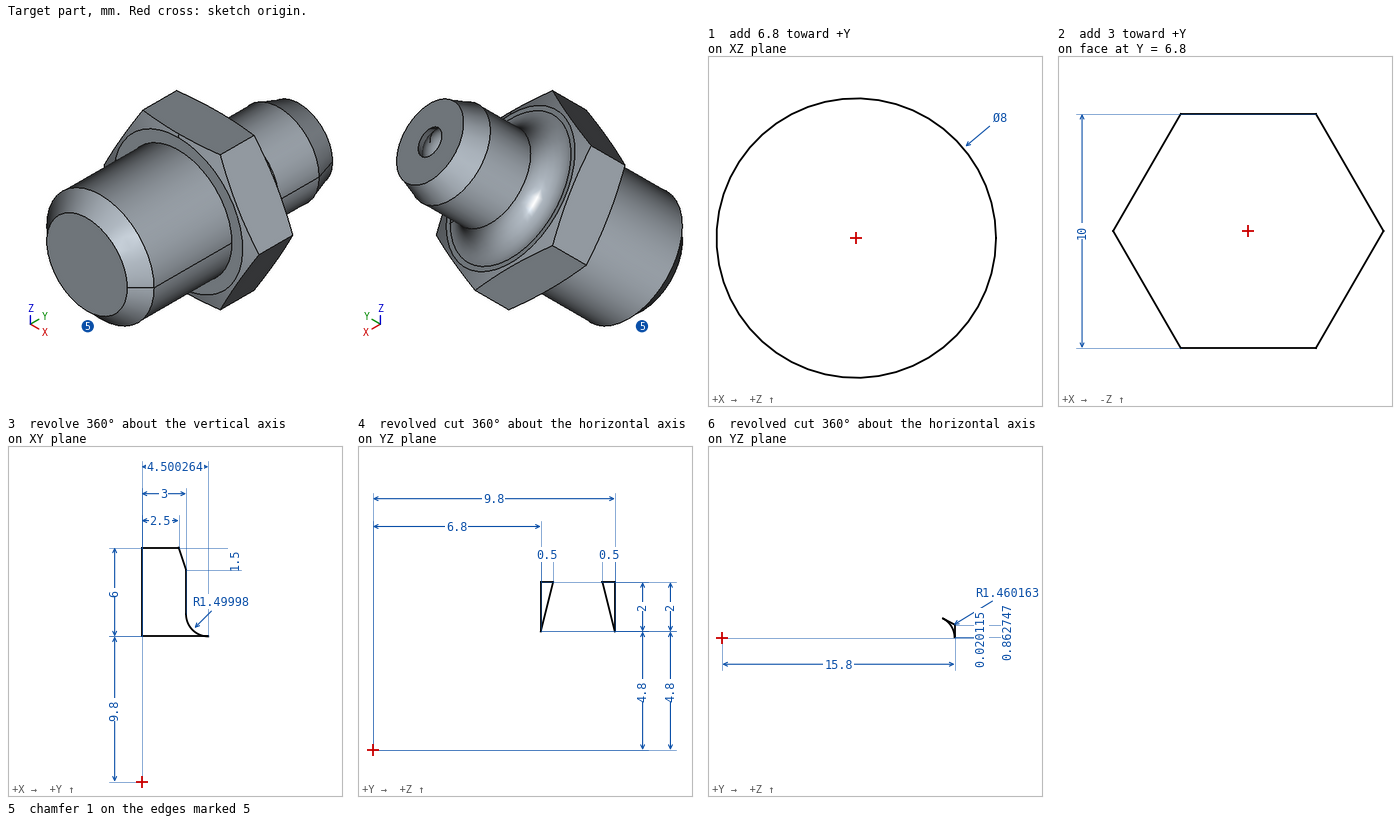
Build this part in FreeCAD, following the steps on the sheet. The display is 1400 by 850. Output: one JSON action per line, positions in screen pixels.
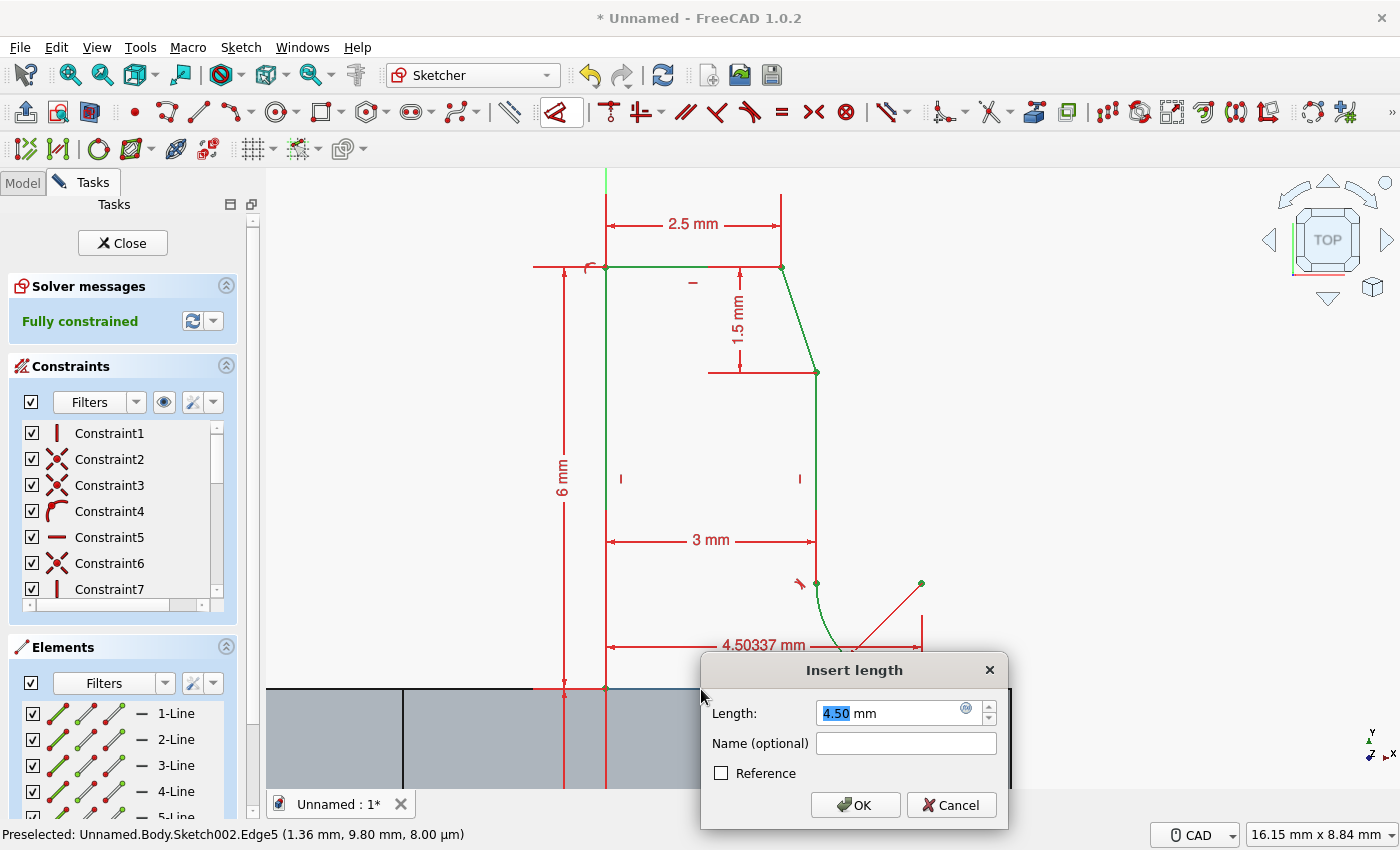
{"action": "type", "text": "4.500264"}
{"action": "key", "text": "Return"}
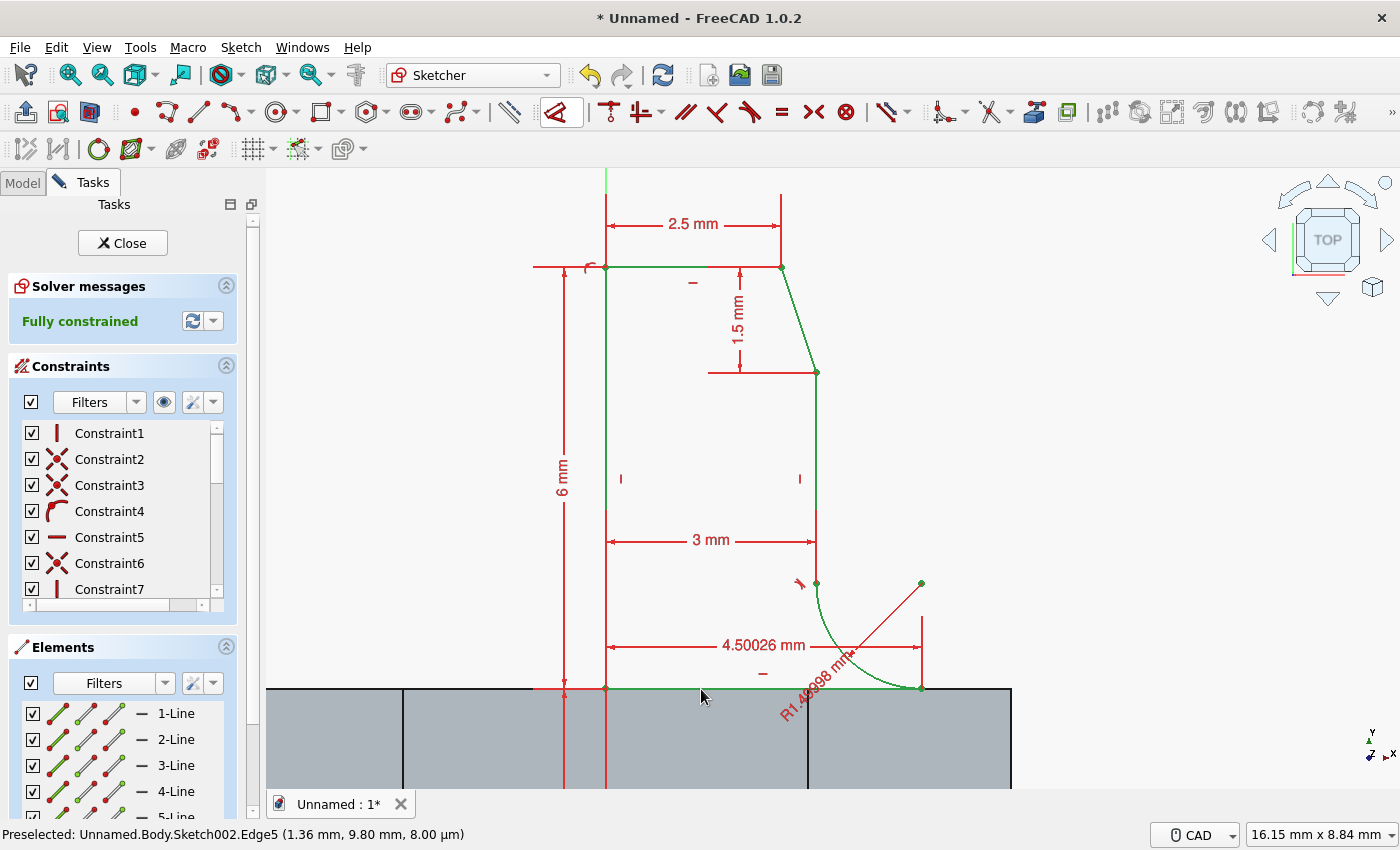
{"action": "left_click", "coordinate": [123, 243]}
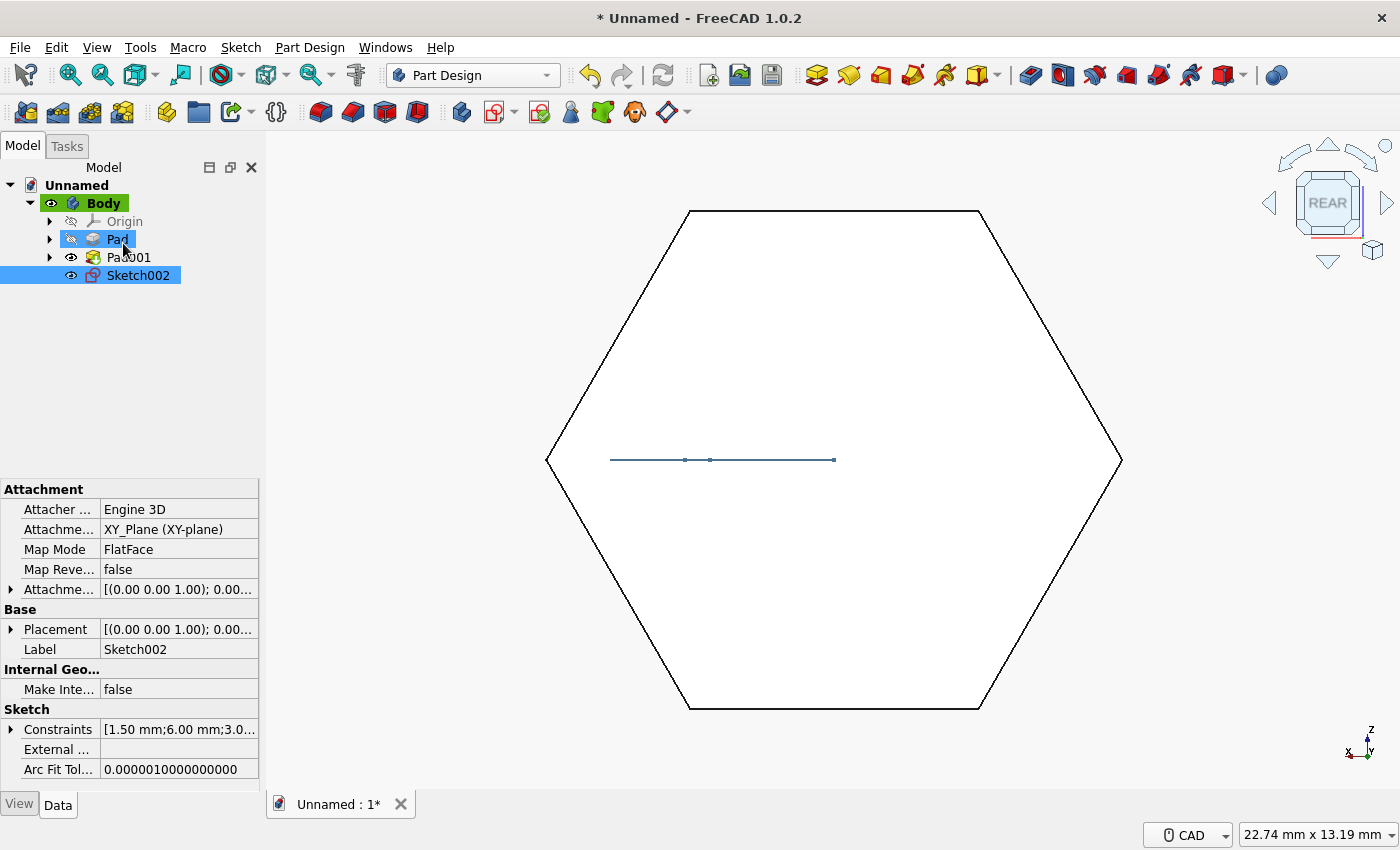
{"action": "left_click", "coordinate": [850, 76]}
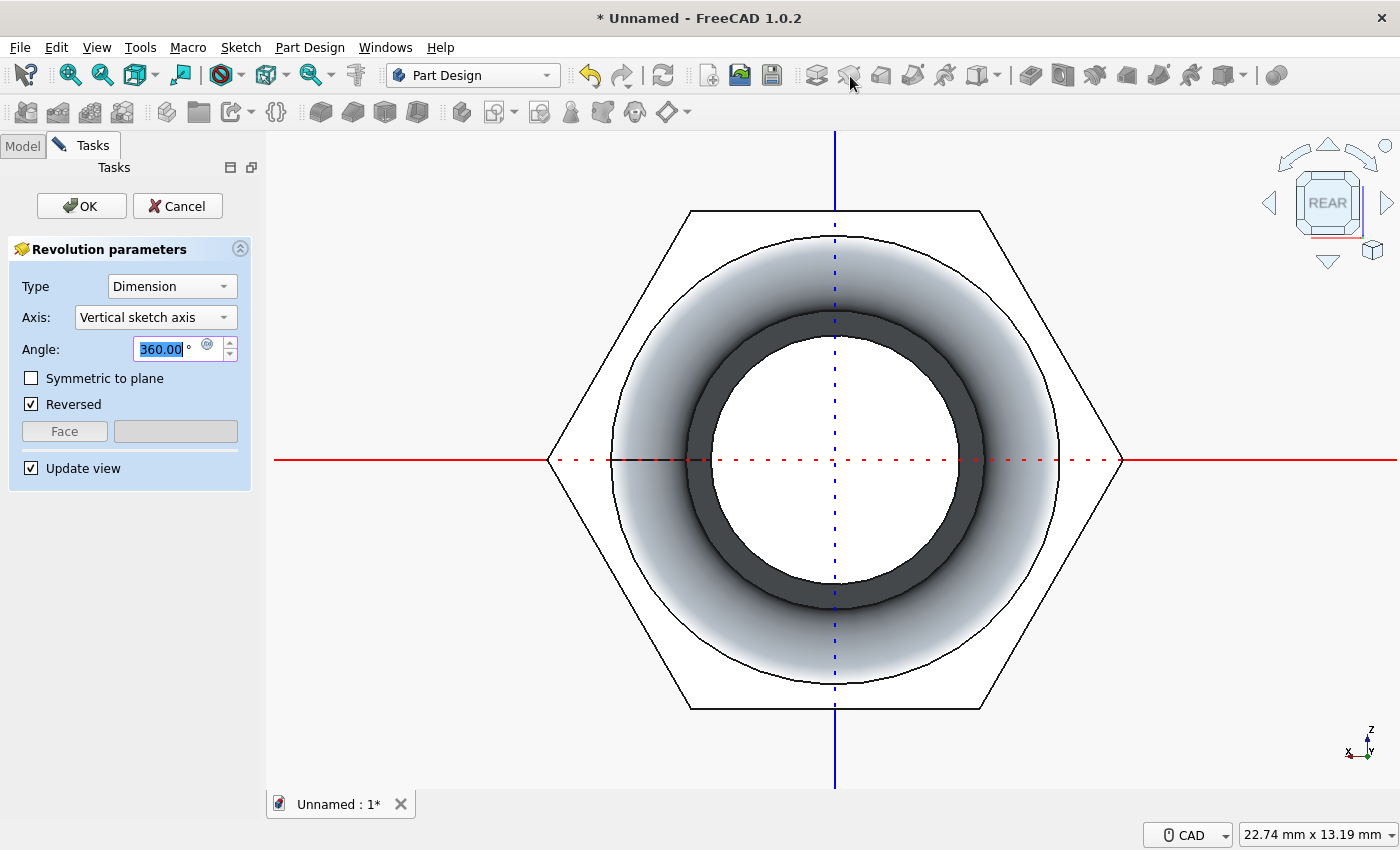
{"action": "left_click", "coordinate": [82, 206]}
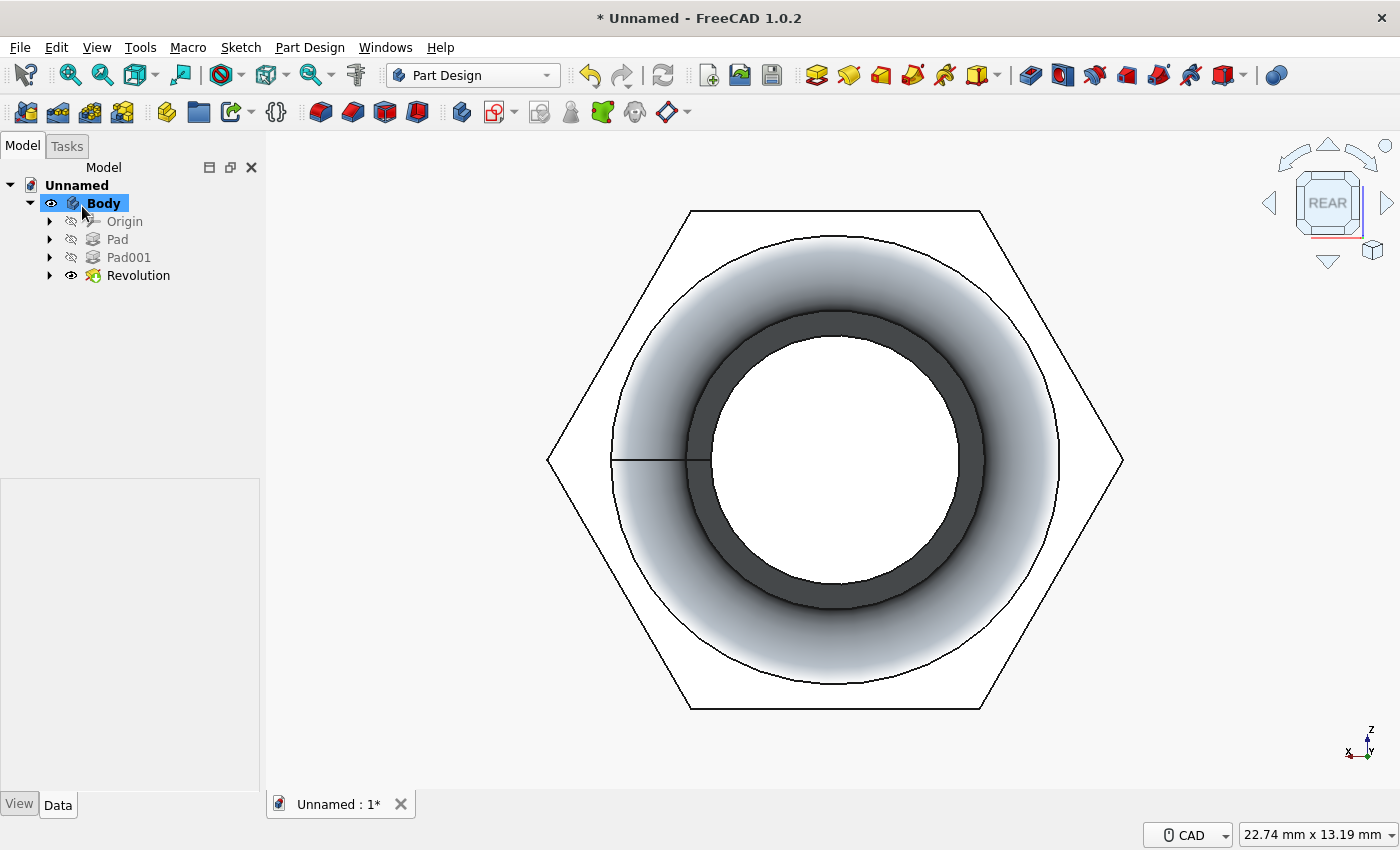
{"action": "left_click", "coordinate": [494, 112]}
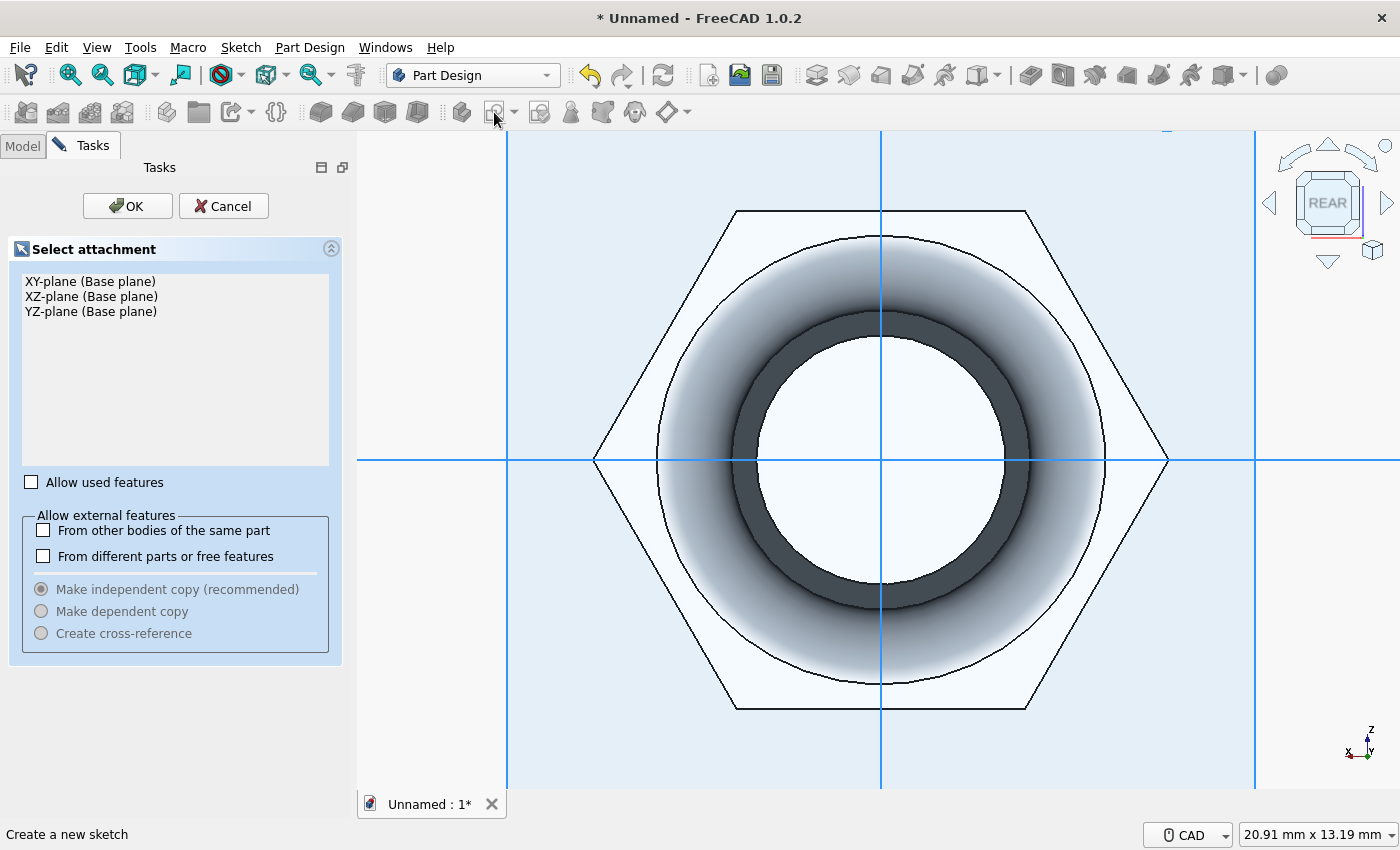
{"action": "left_click", "coordinate": [82, 312]}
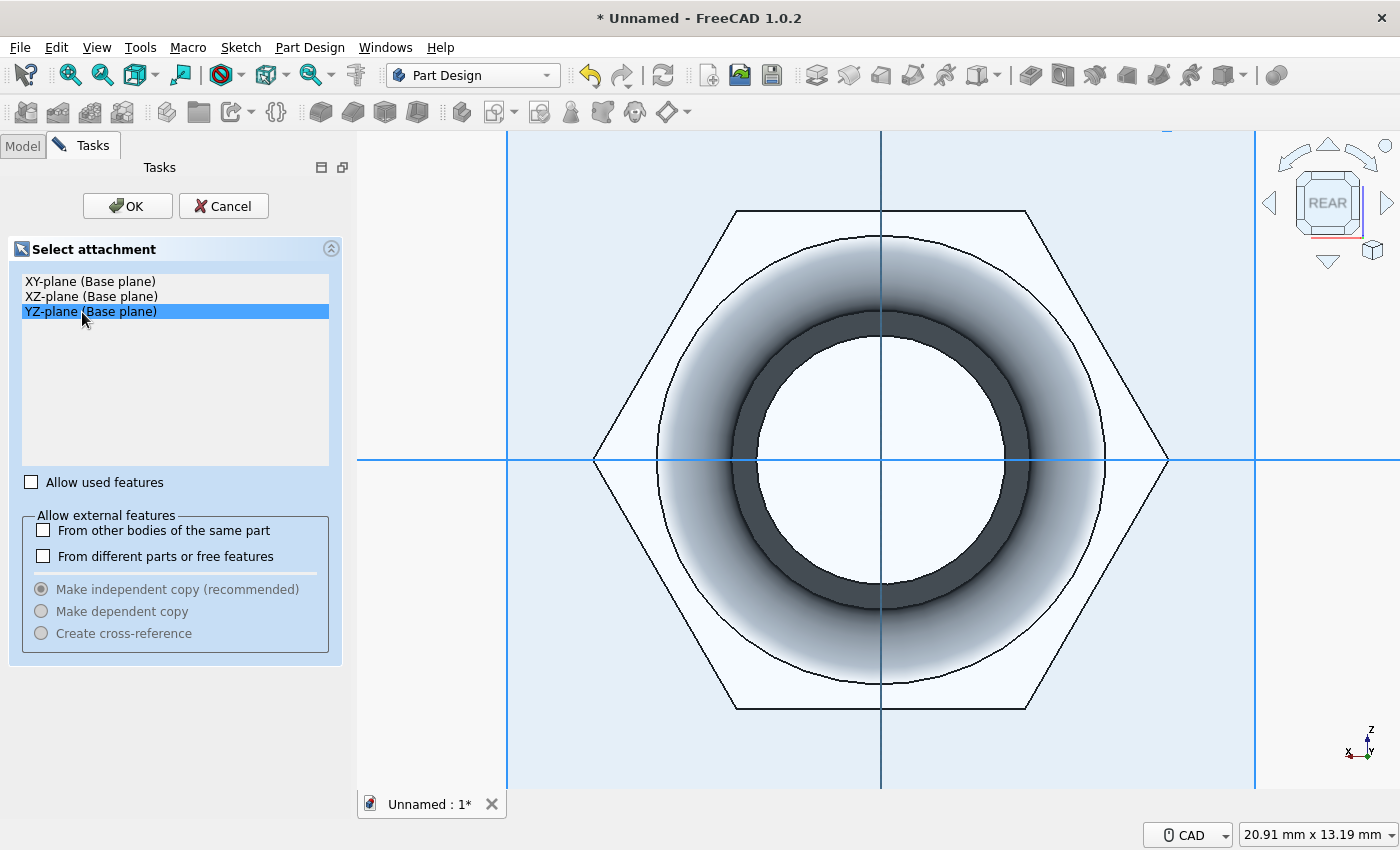
{"action": "left_click", "coordinate": [128, 206]}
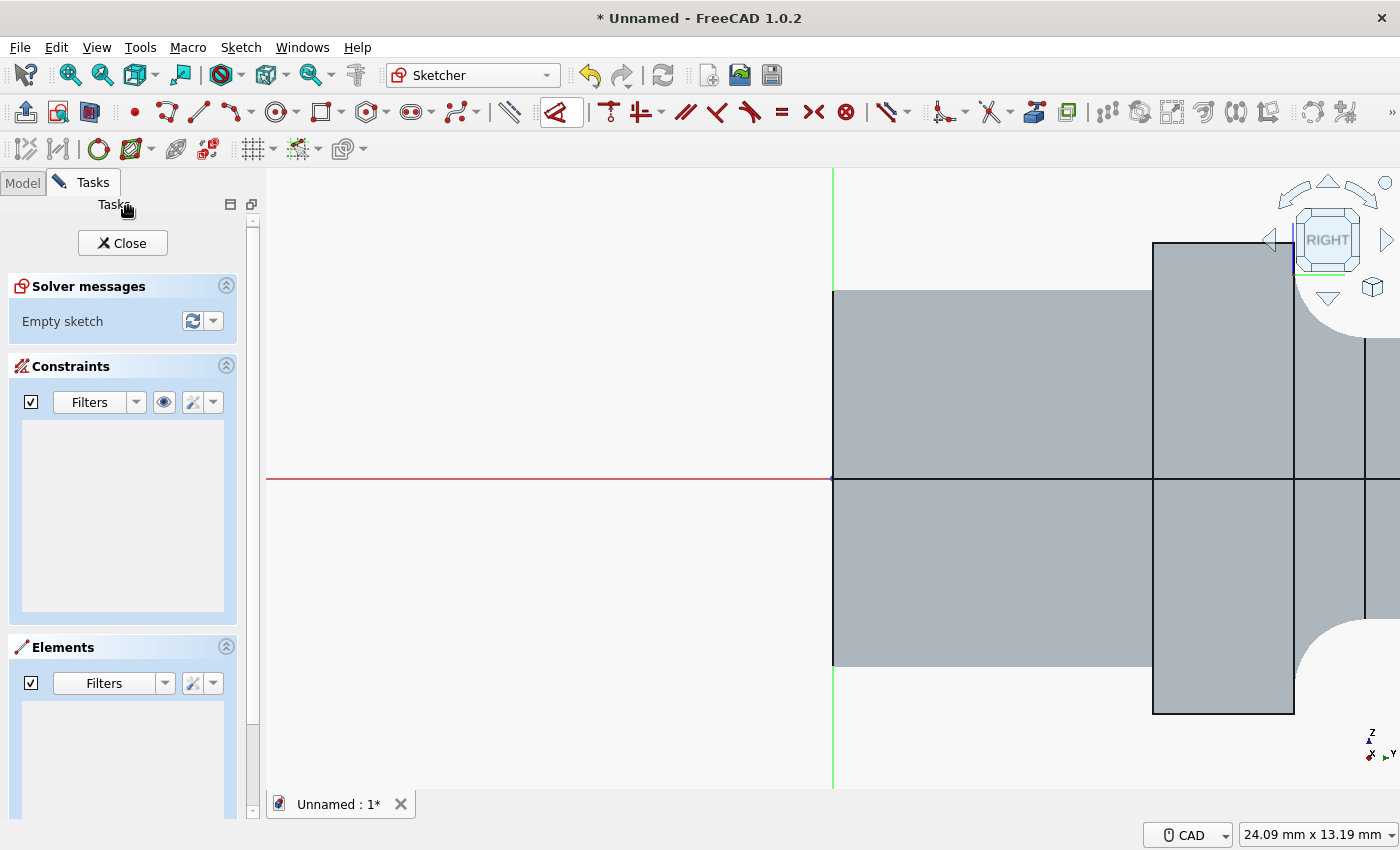
{"action": "key", "text": "q s"}